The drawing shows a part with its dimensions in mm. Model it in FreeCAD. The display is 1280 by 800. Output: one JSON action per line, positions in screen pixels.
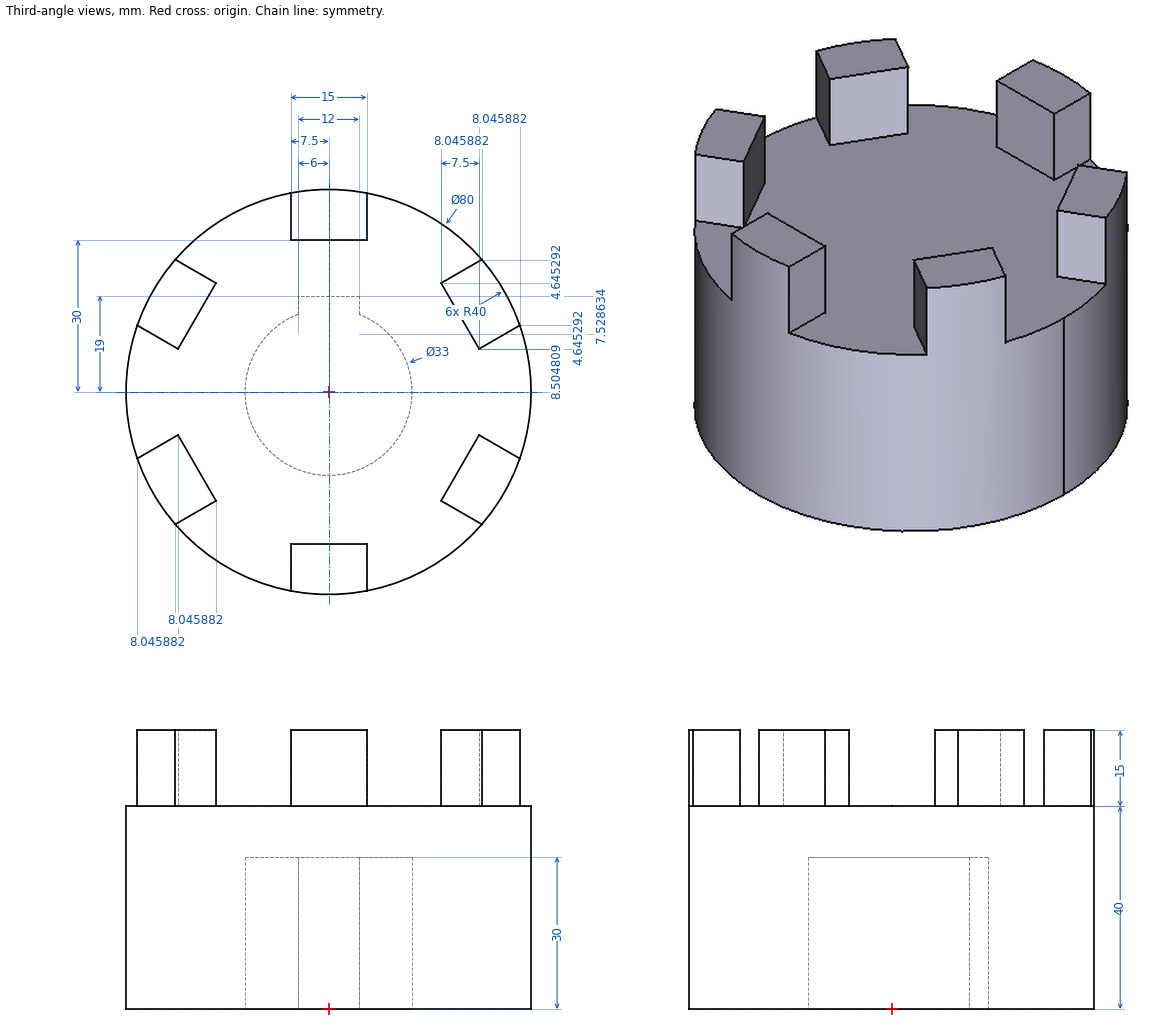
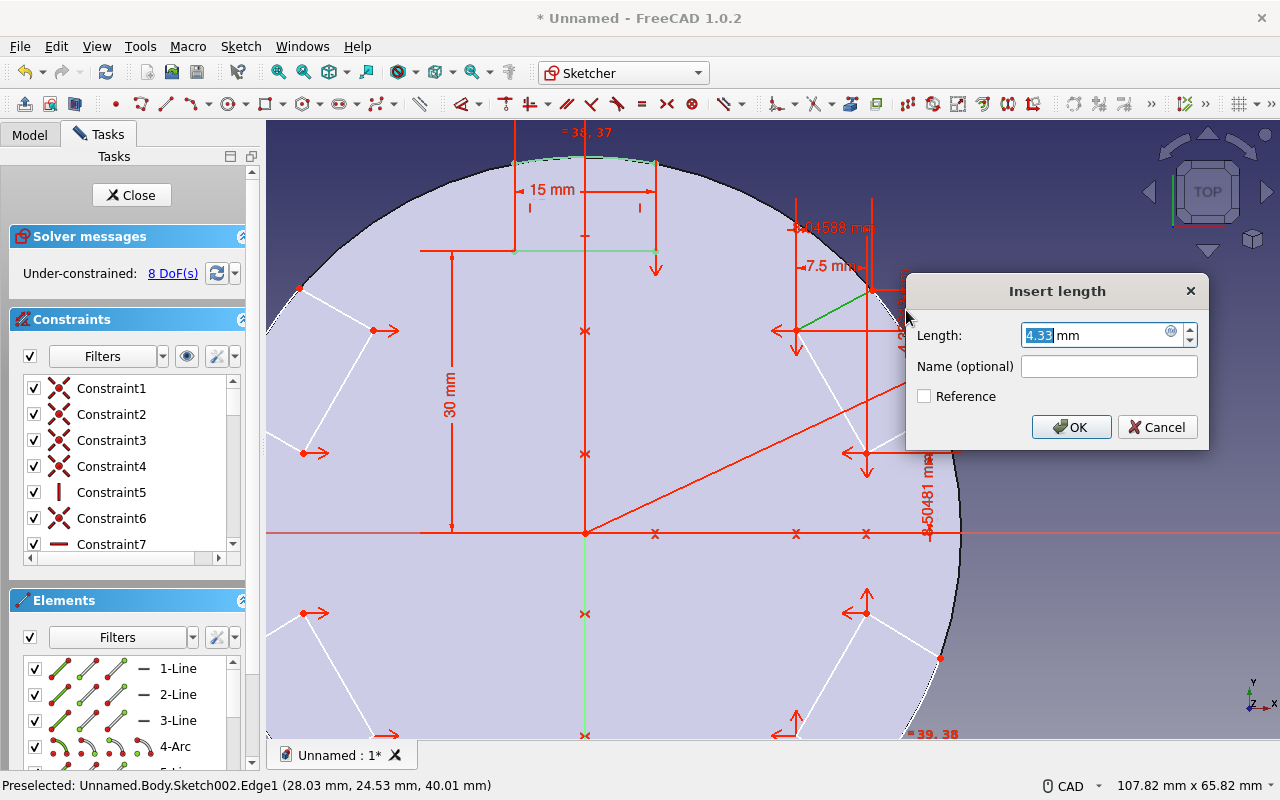
{"action": "type", "text": "4.645292"}
{"action": "key", "text": "Return"}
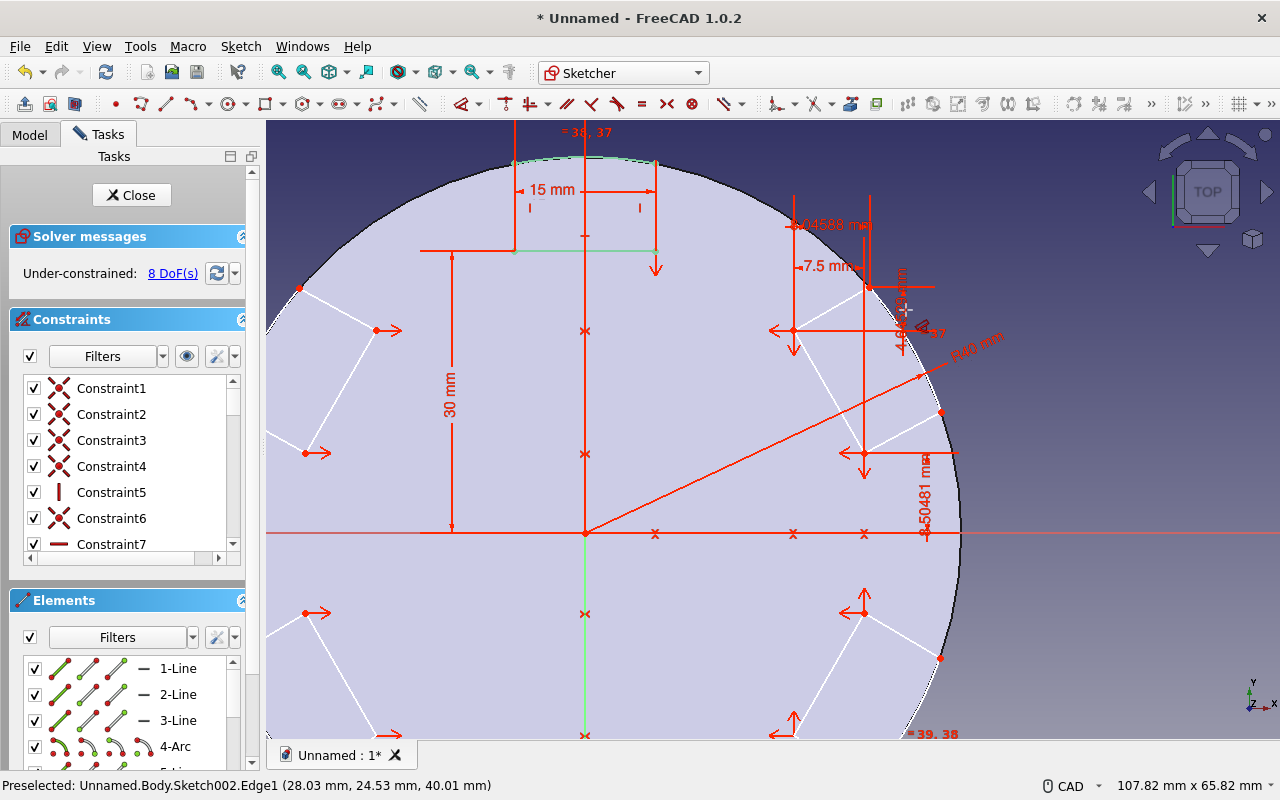
{"action": "left_click", "coordinate": [888, 441]}
{"action": "left_click", "coordinate": [903, 378]}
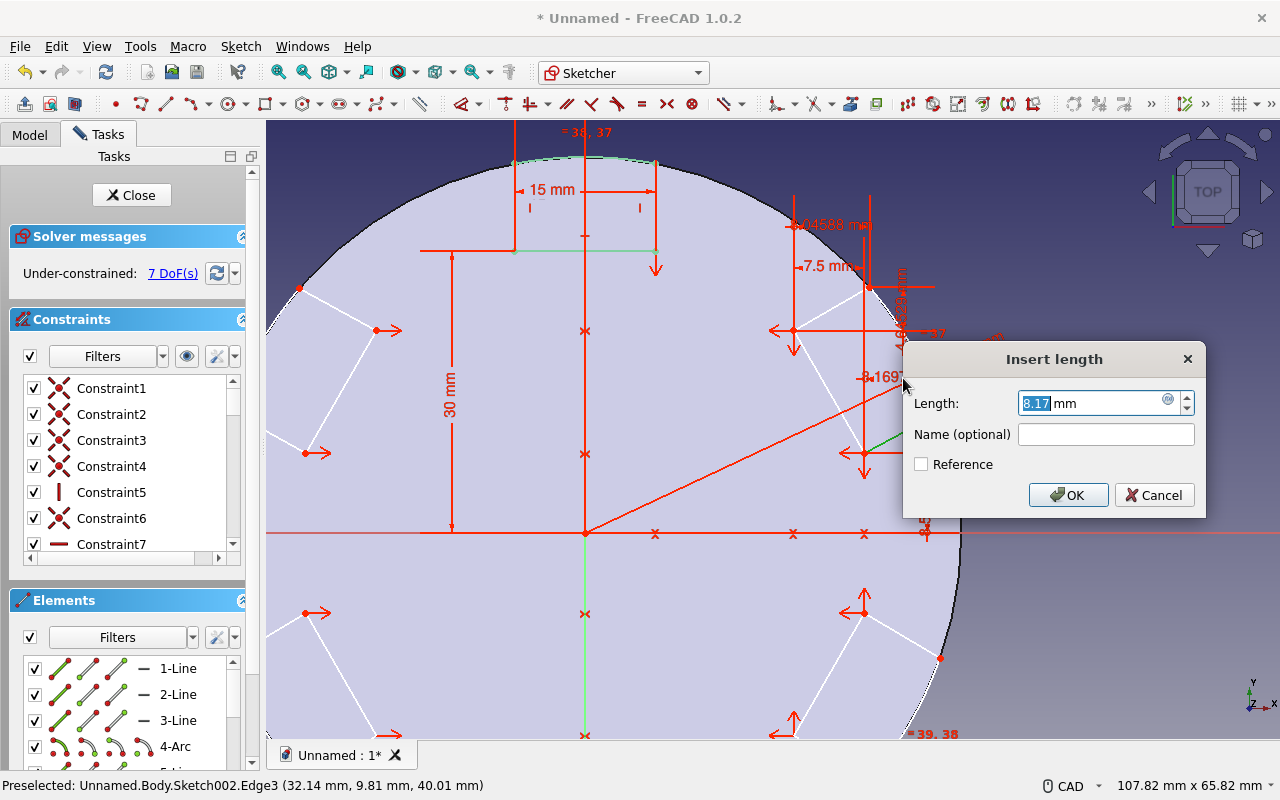
{"action": "type", "text": "8.045882"}
{"action": "key", "text": "Return"}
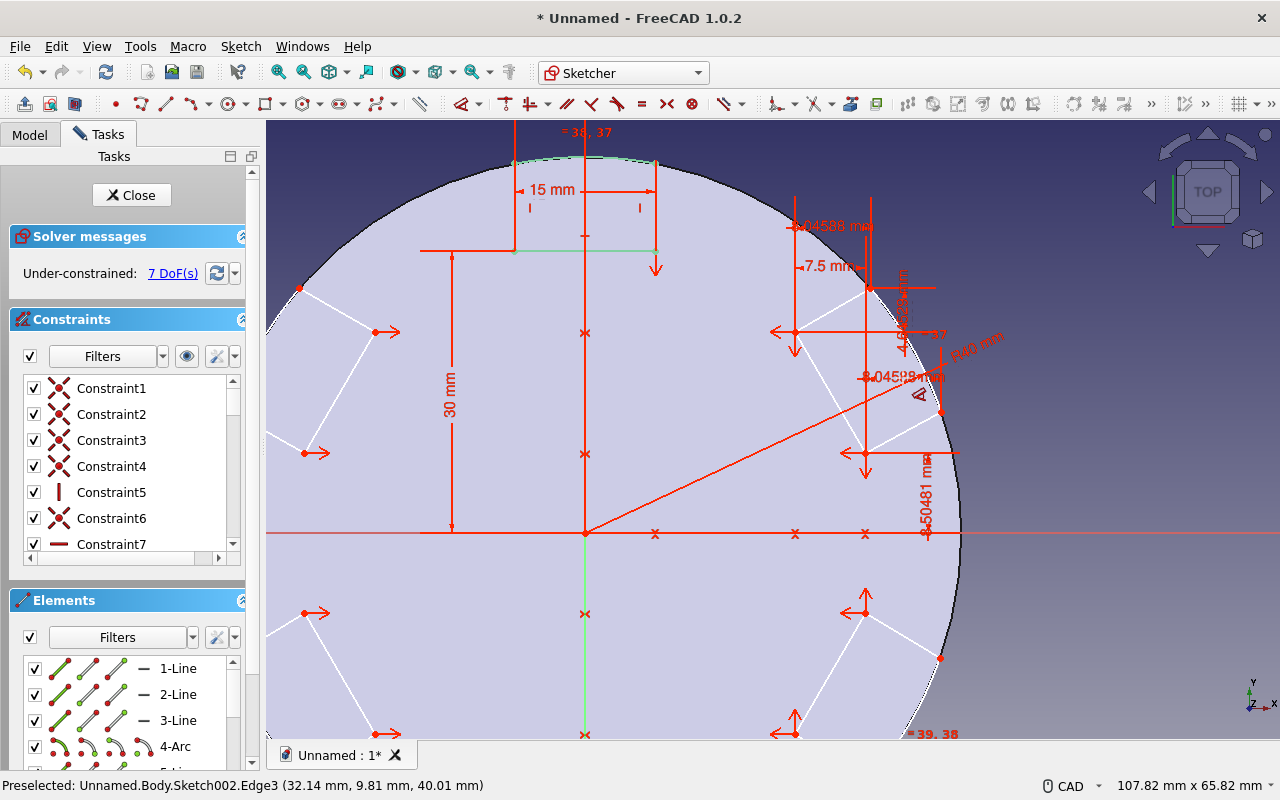
{"action": "left_click", "coordinate": [888, 441]}
{"action": "left_click", "coordinate": [975, 433]}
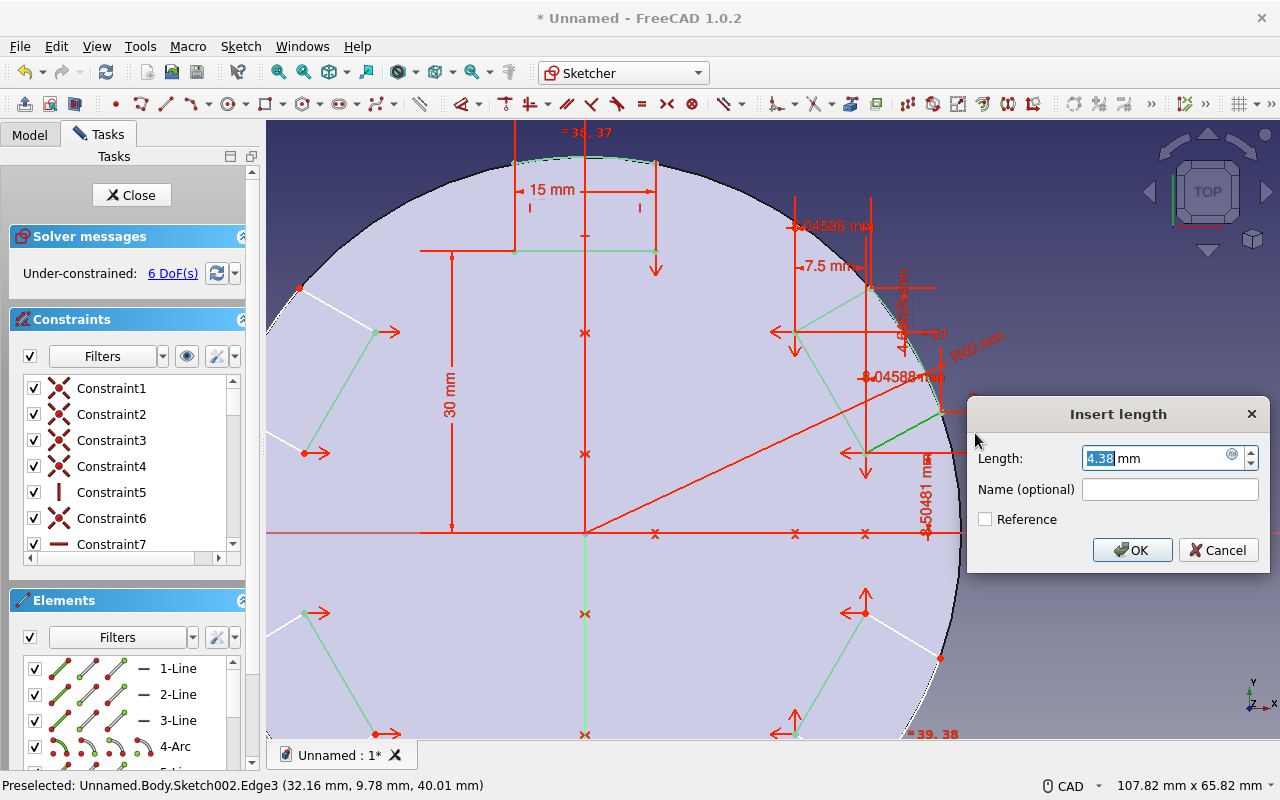
{"action": "type", "text": "4.645292"}
{"action": "key", "text": "Return"}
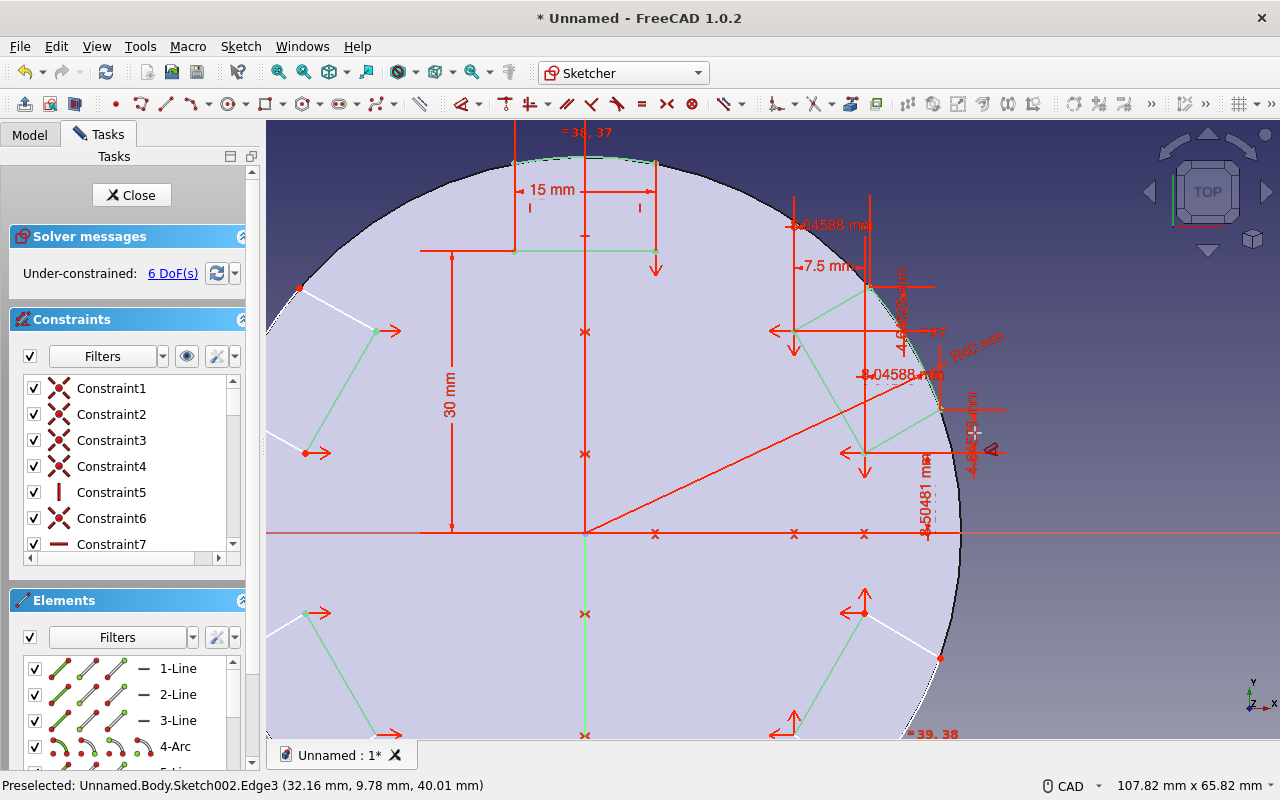
{"action": "left_click", "coordinate": [917, 645]}
{"action": "left_click", "coordinate": [902, 692]}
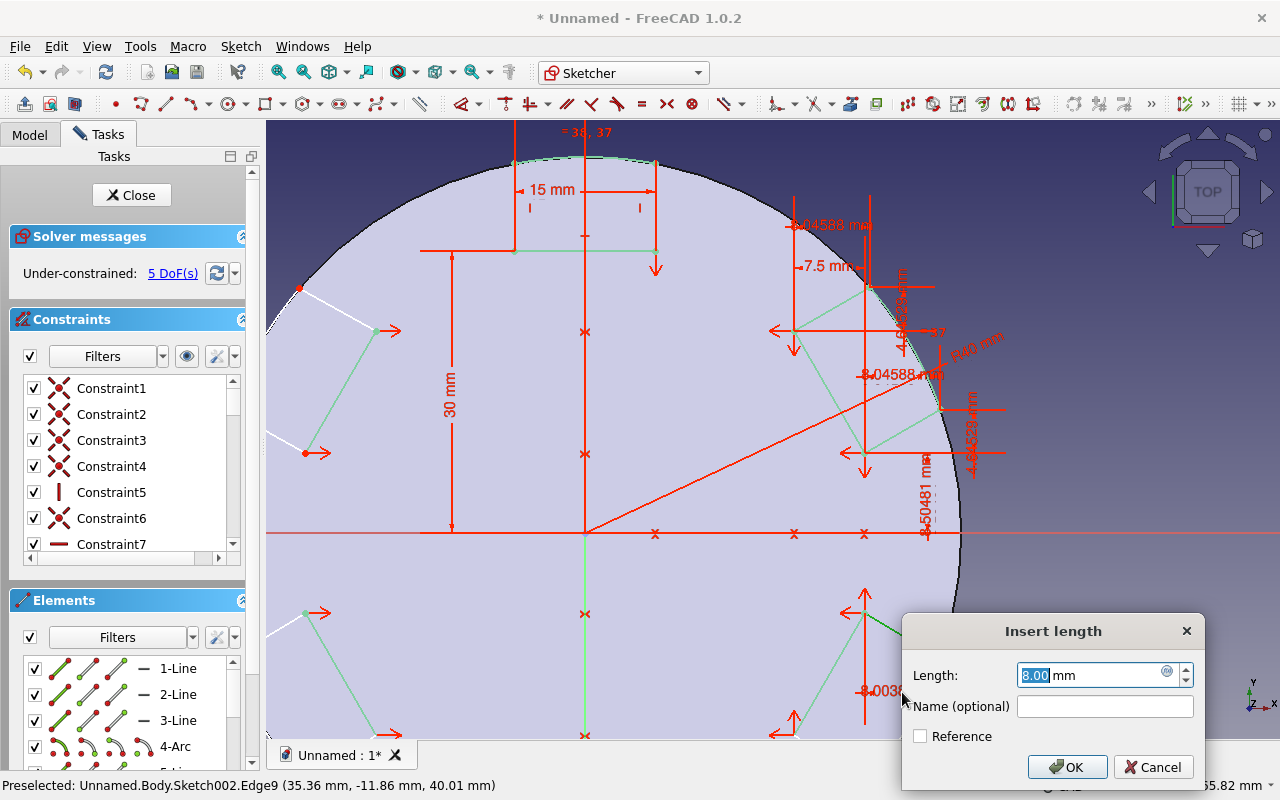
{"action": "type", "text": "8.045882"}
{"action": "key", "text": "Return"}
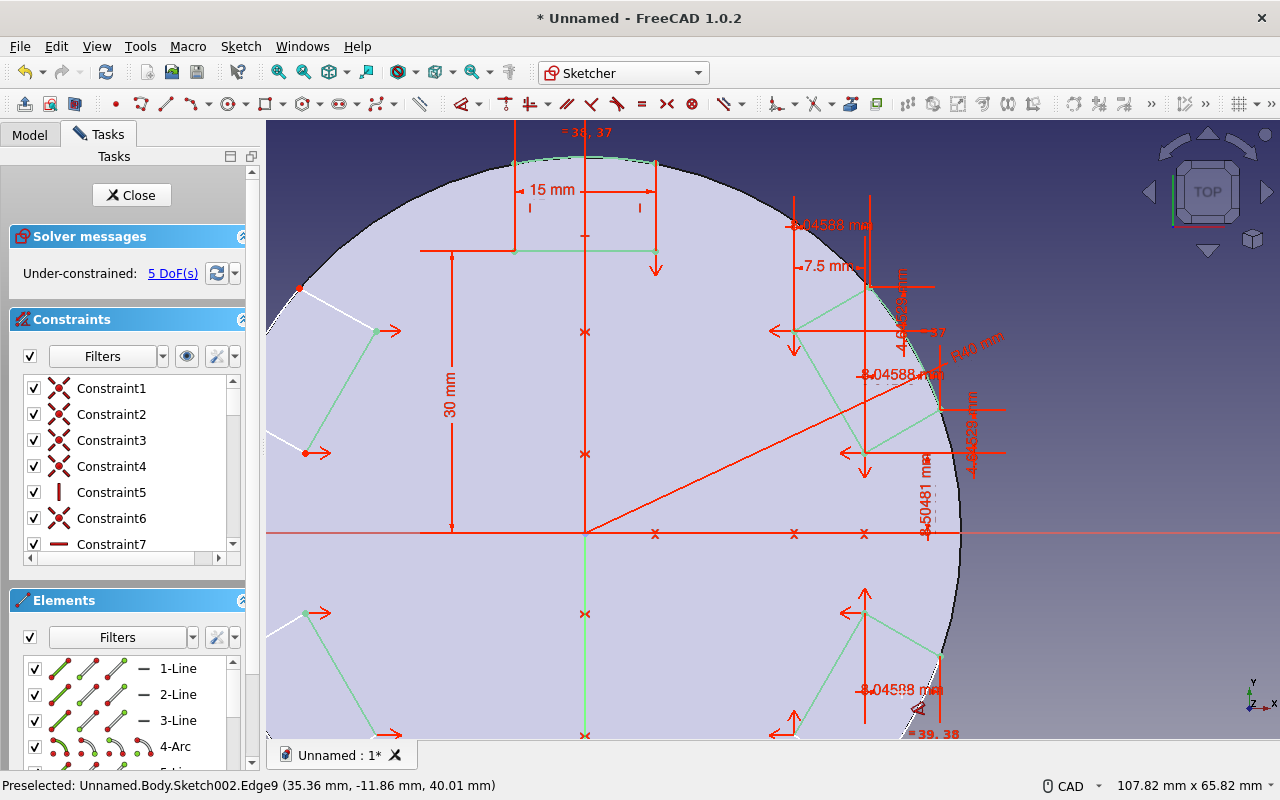
{"action": "scroll", "coordinate": [850, 303], "scroll_direction": "down", "scroll_amount": 3}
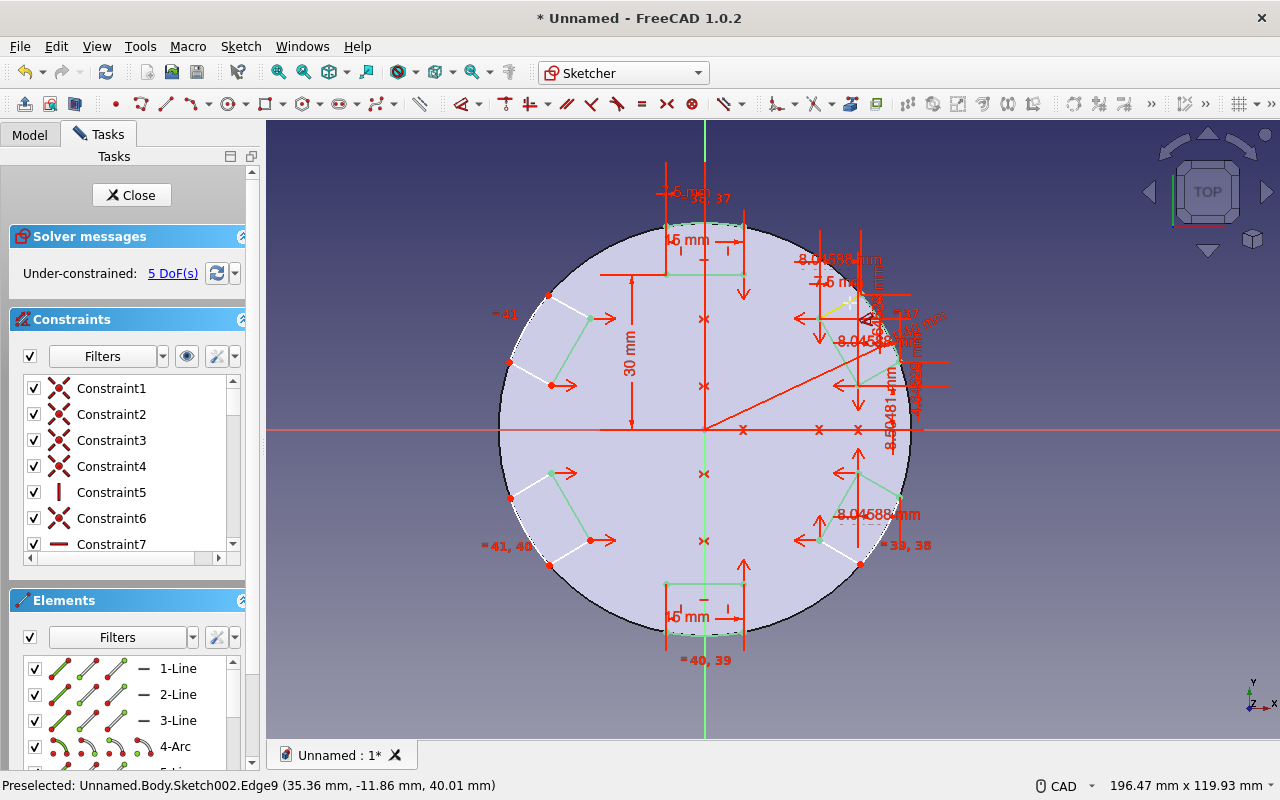
{"action": "left_click", "coordinate": [832, 548]}
{"action": "left_click", "coordinate": [840, 599]}